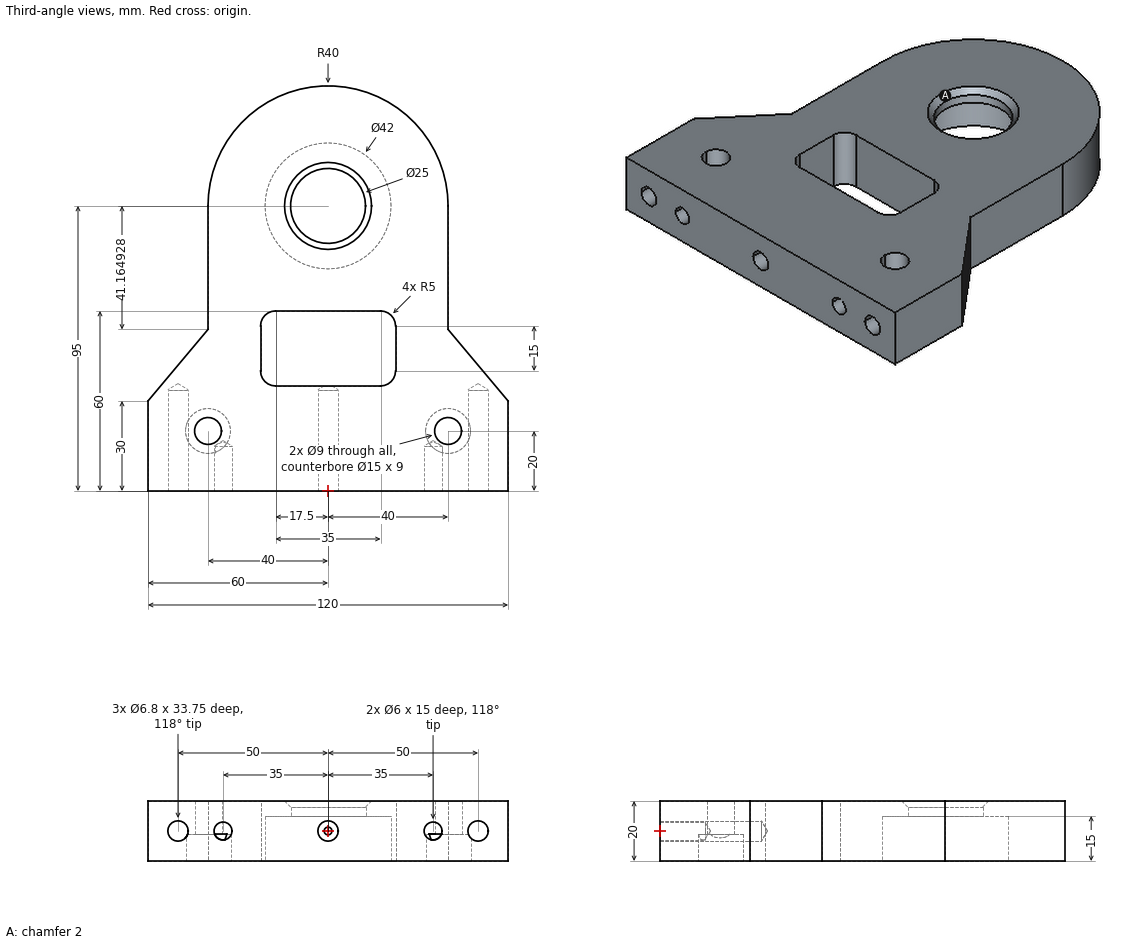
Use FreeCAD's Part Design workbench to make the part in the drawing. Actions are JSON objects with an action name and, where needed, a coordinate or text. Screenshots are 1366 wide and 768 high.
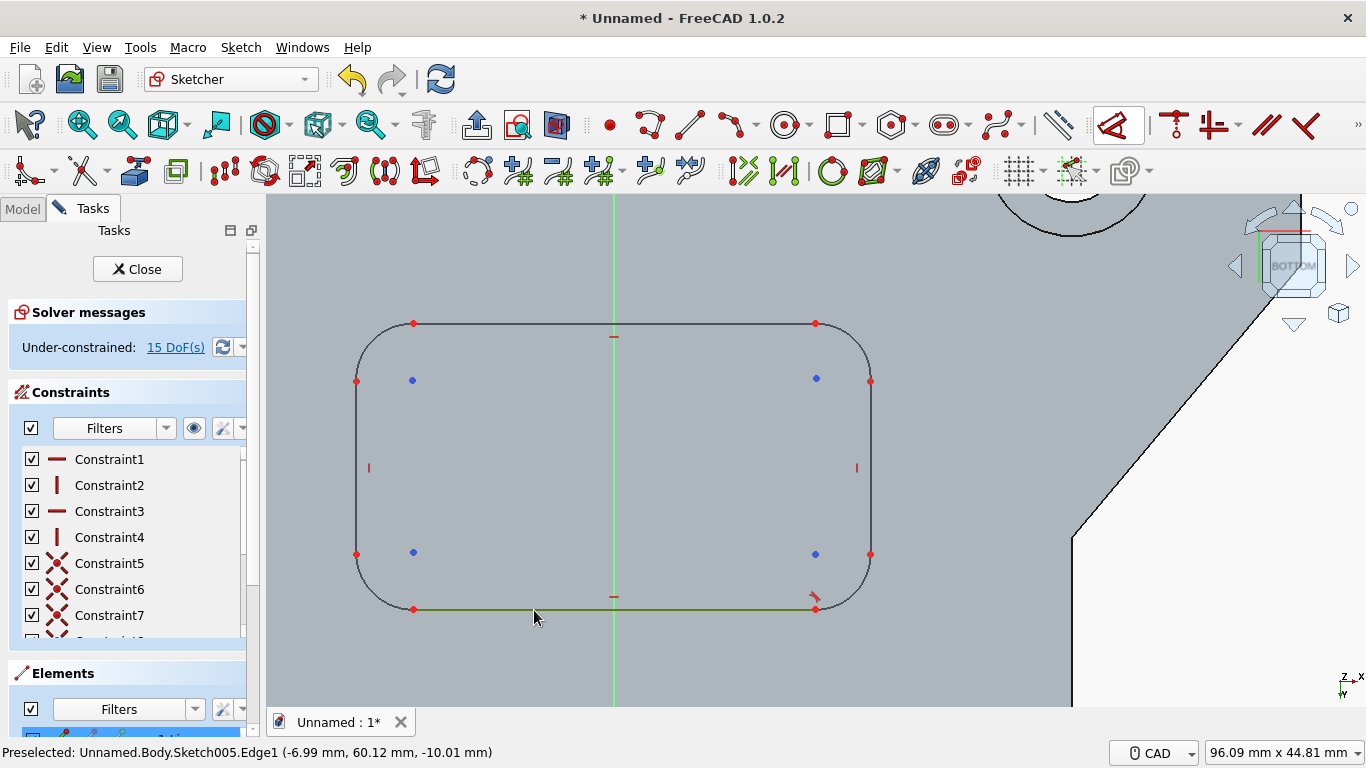
{"action": "left_click", "coordinate": [363, 580]}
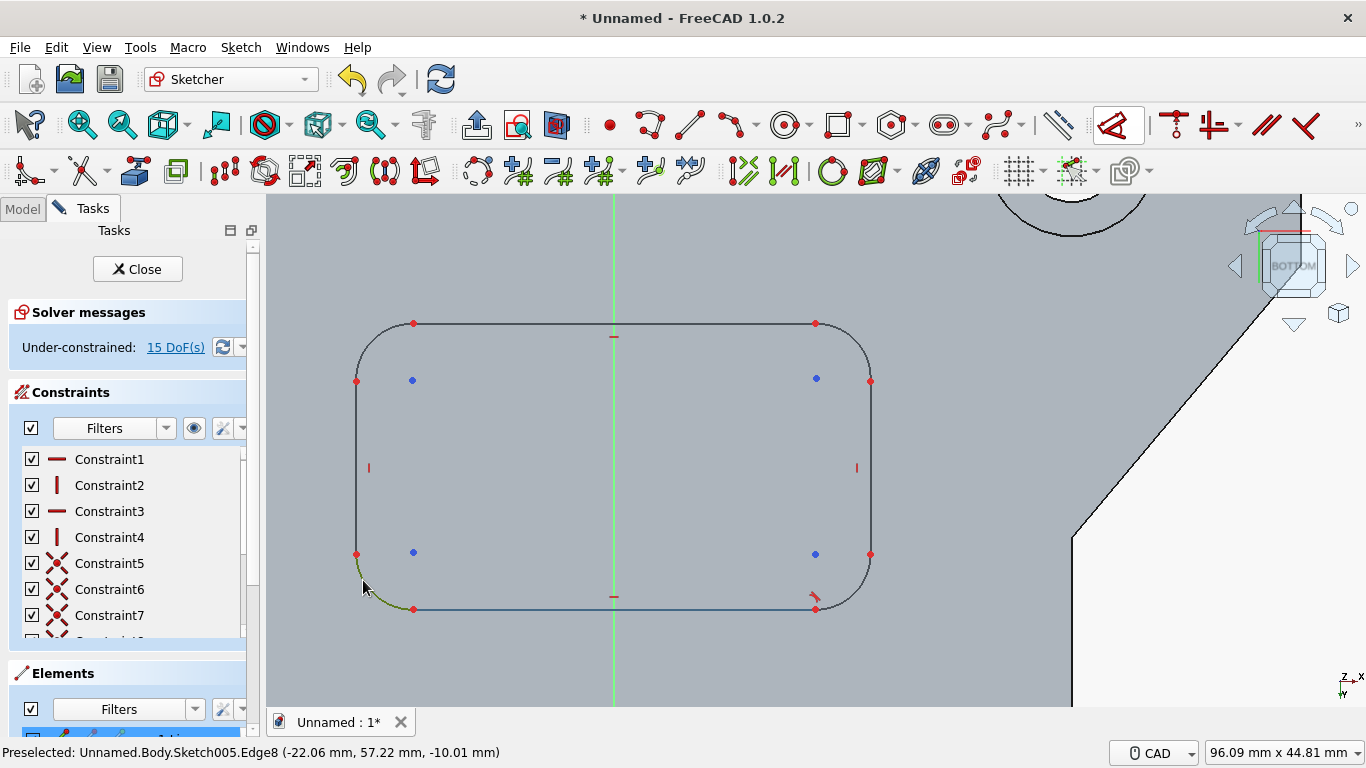
{"action": "key", "text": "t"}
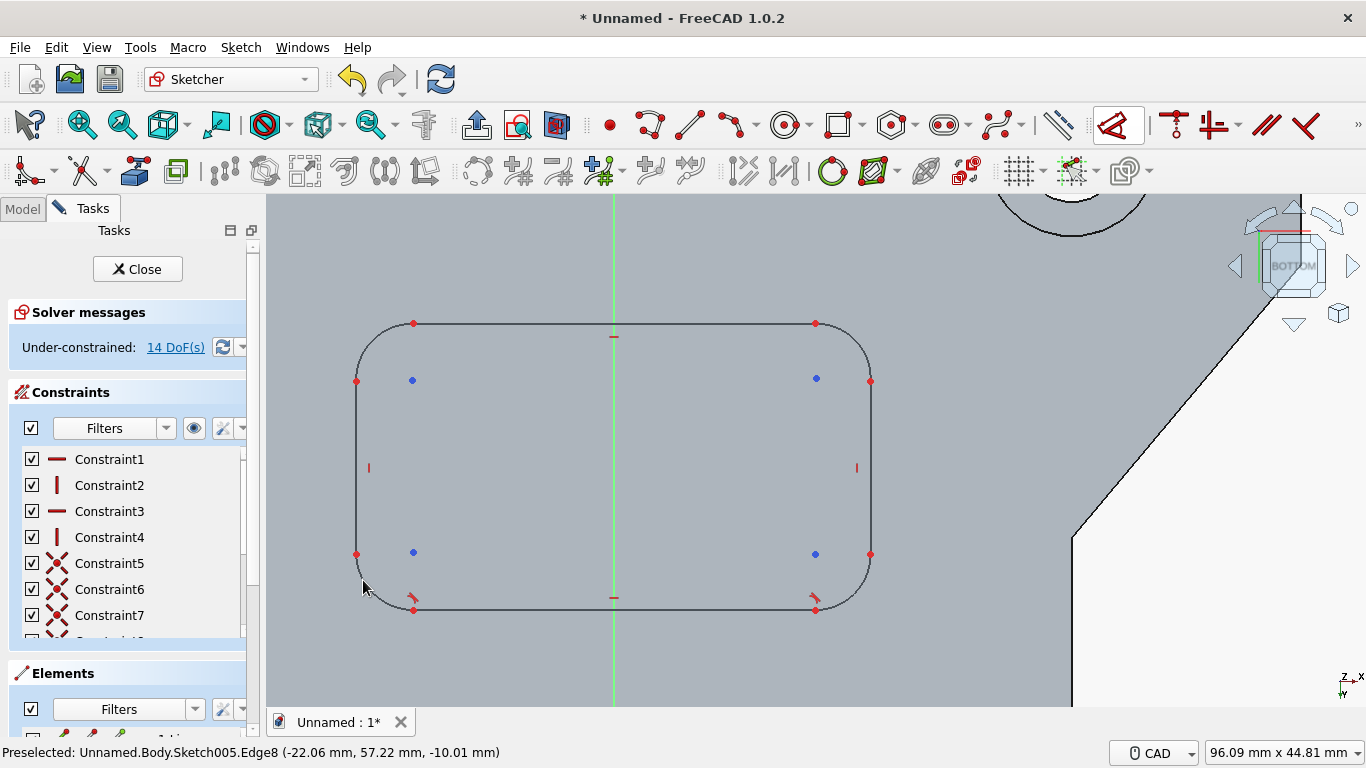
{"action": "left_click", "coordinate": [871, 502]}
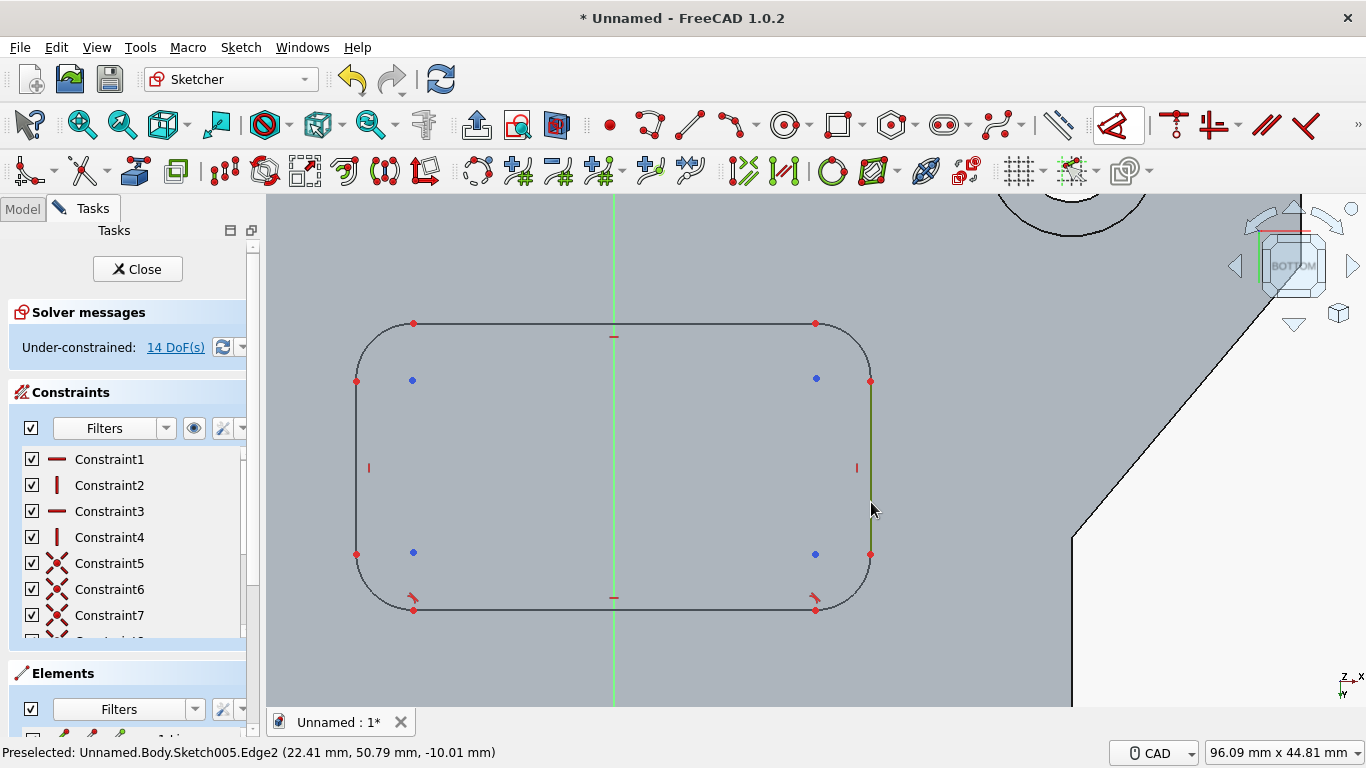
{"action": "left_click", "coordinate": [840, 604]}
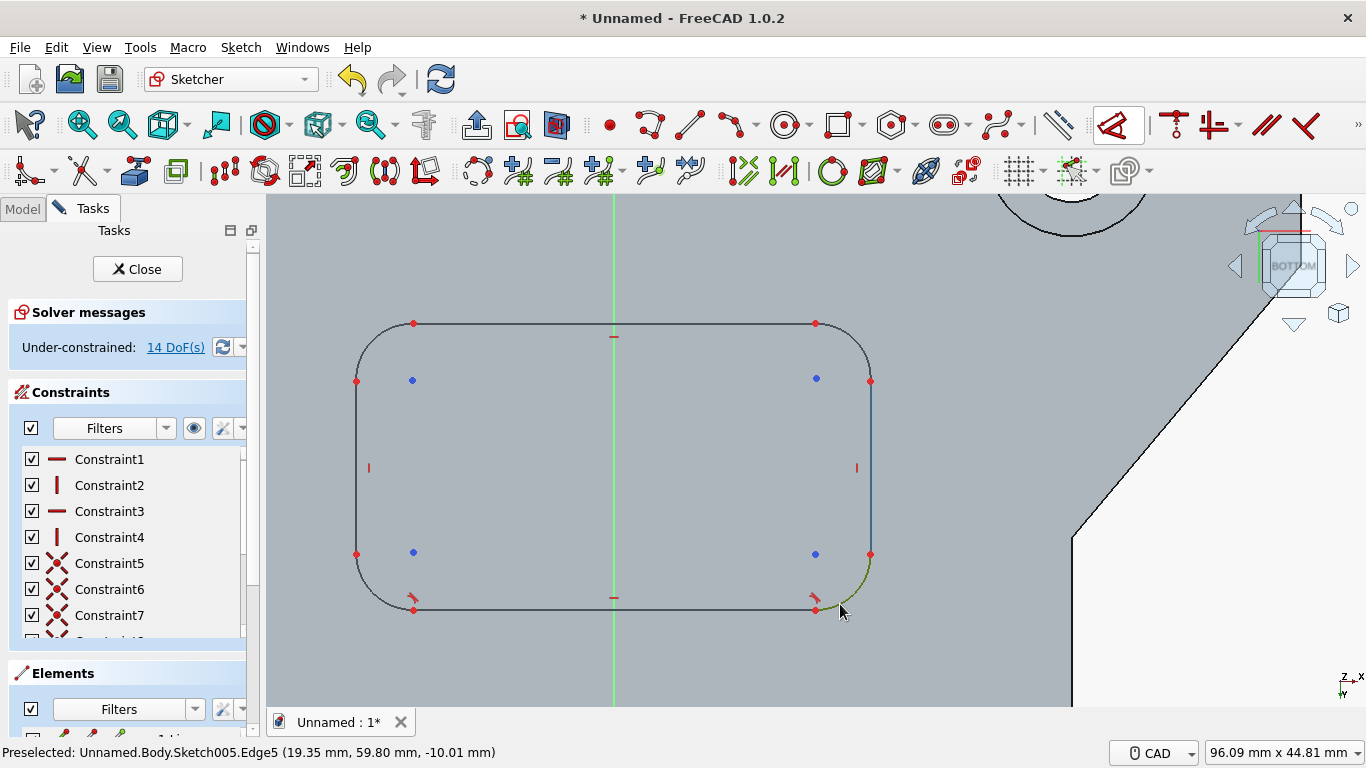
{"action": "key", "text": "t"}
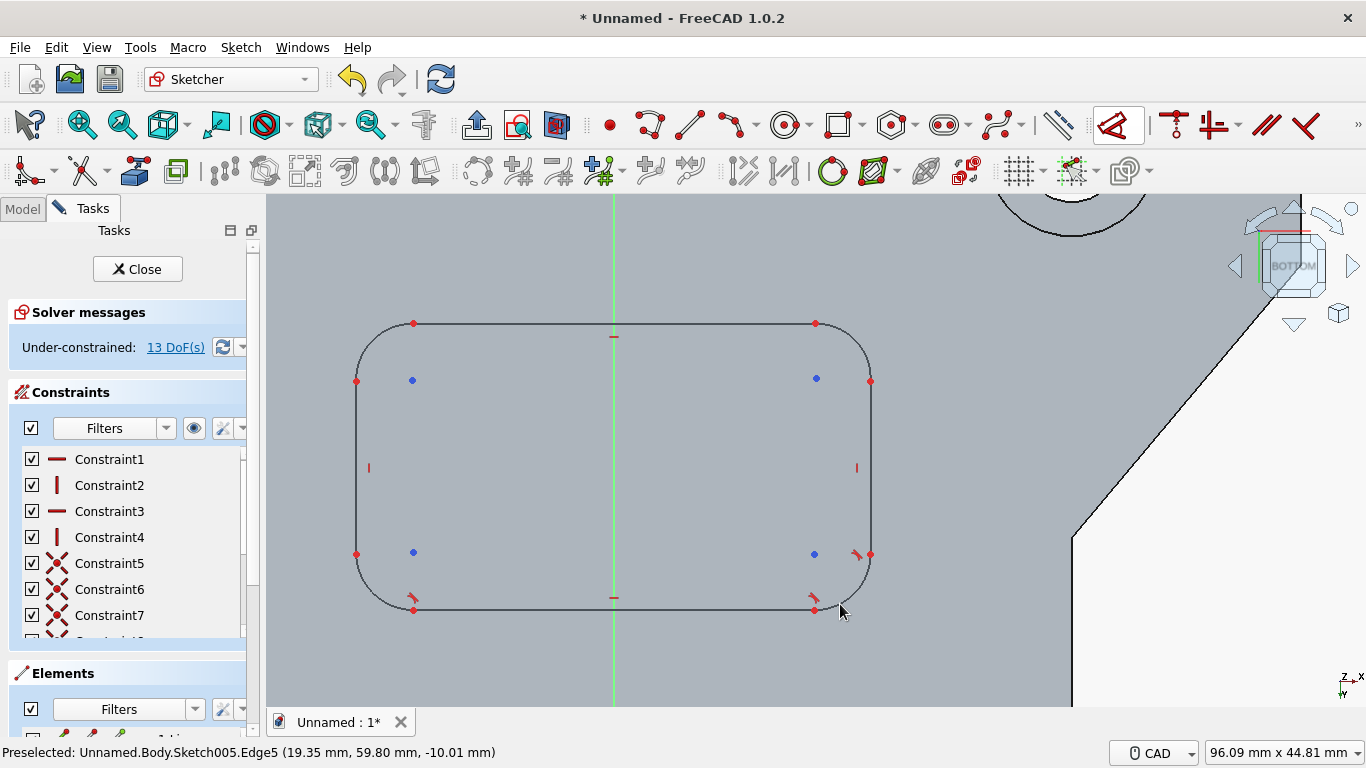
{"action": "left_click", "coordinate": [871, 502]}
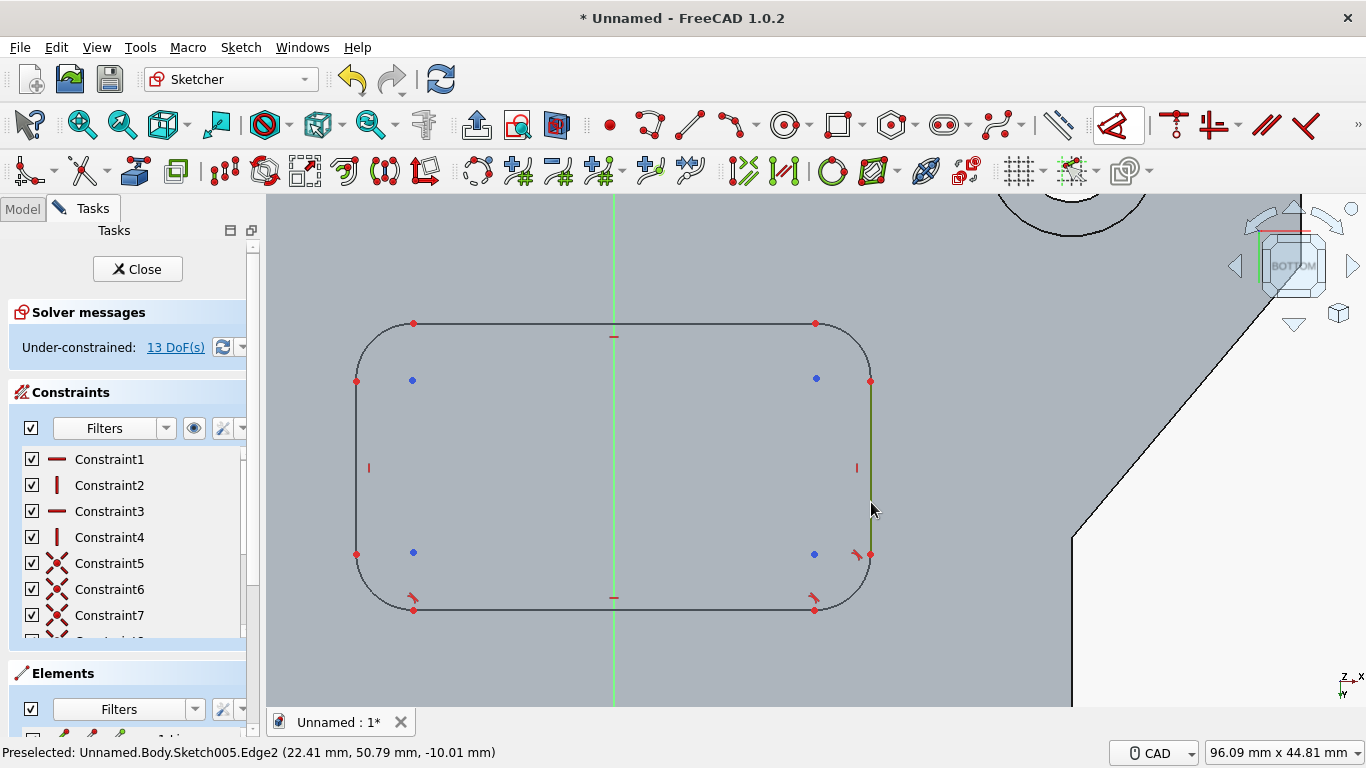
{"action": "left_click", "coordinate": [866, 355]}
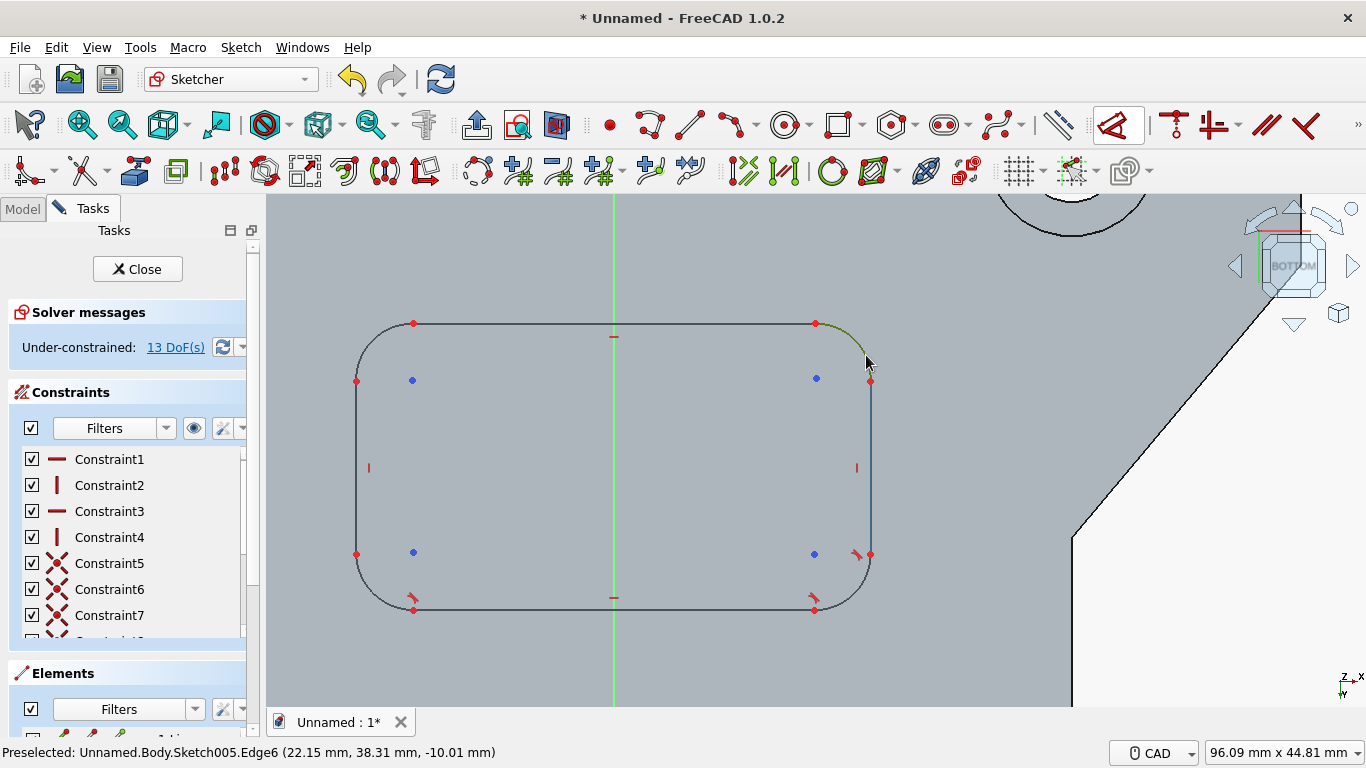
{"action": "key", "text": "t"}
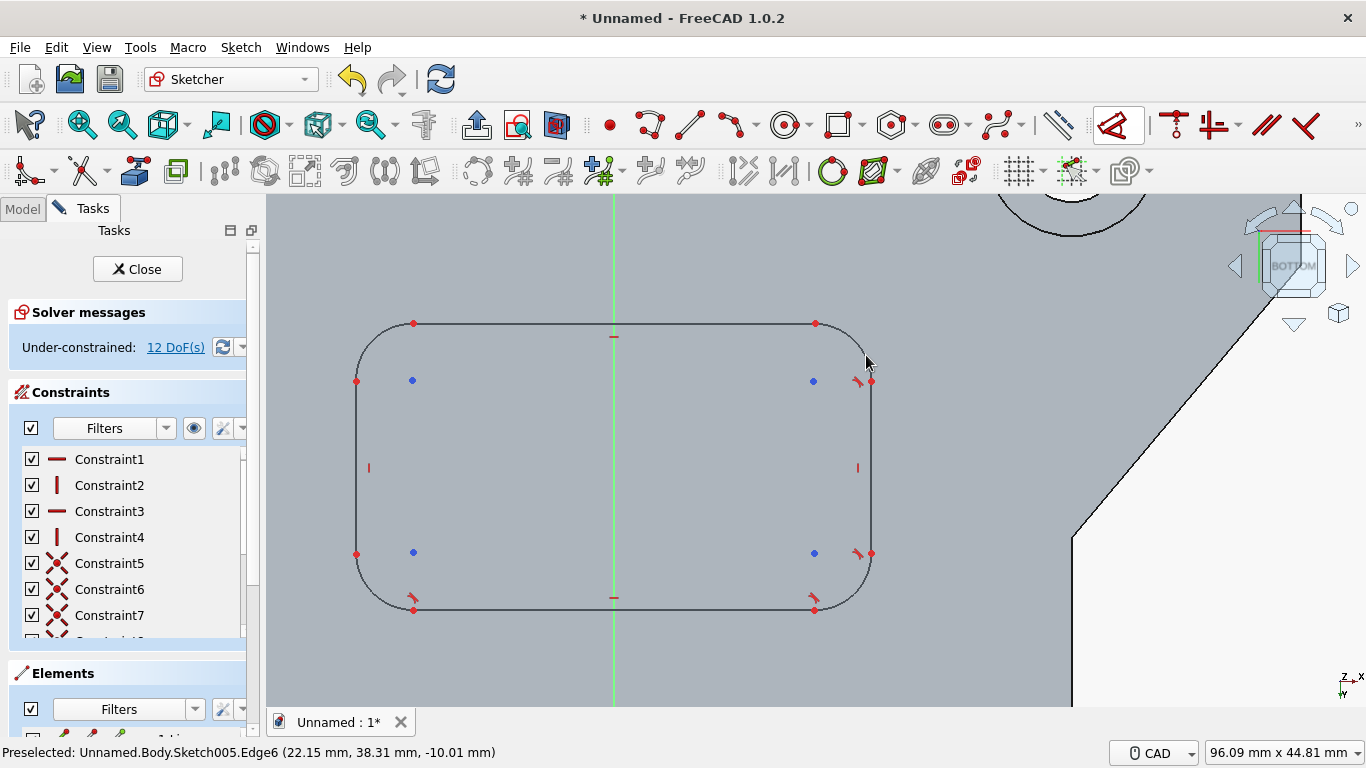
{"action": "left_click", "coordinate": [695, 324]}